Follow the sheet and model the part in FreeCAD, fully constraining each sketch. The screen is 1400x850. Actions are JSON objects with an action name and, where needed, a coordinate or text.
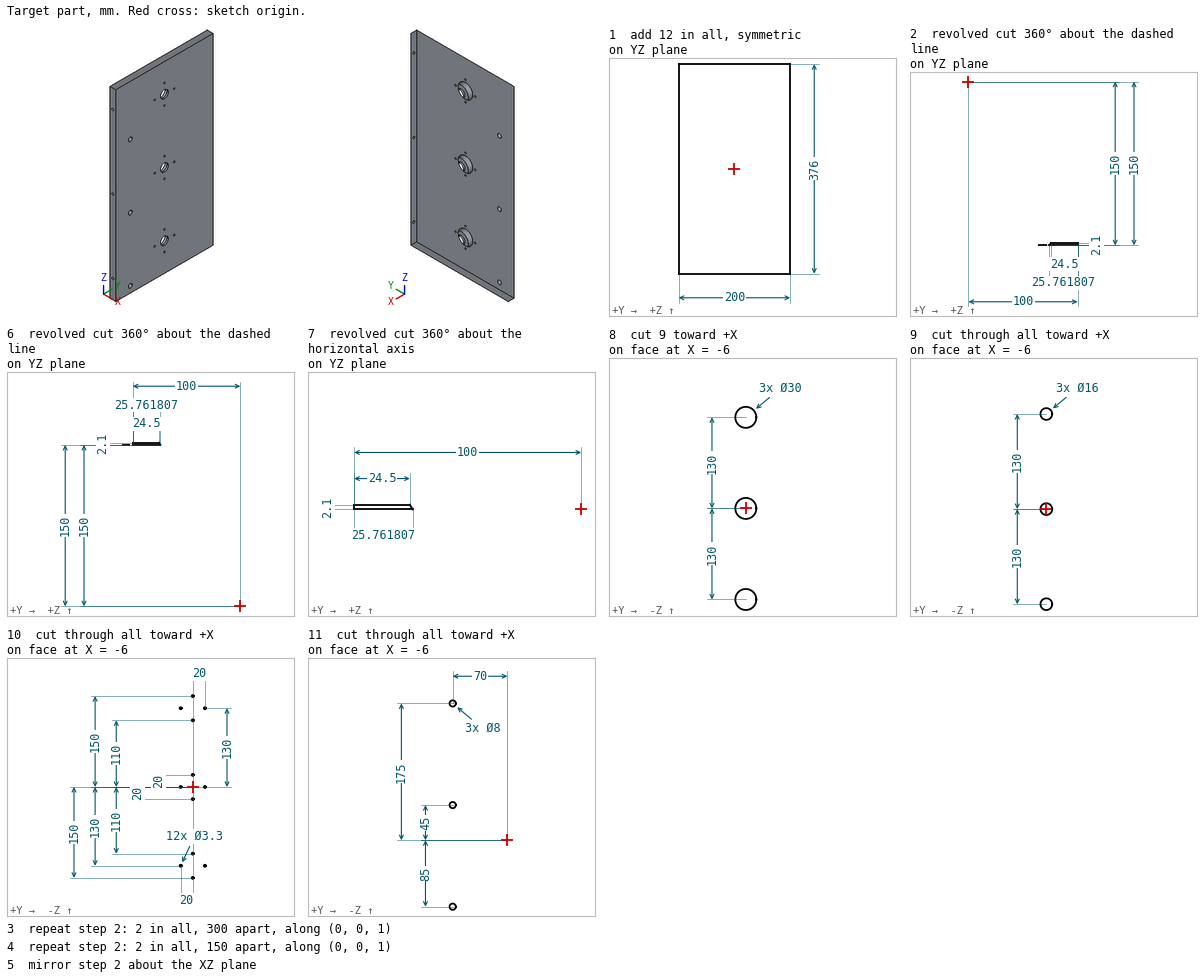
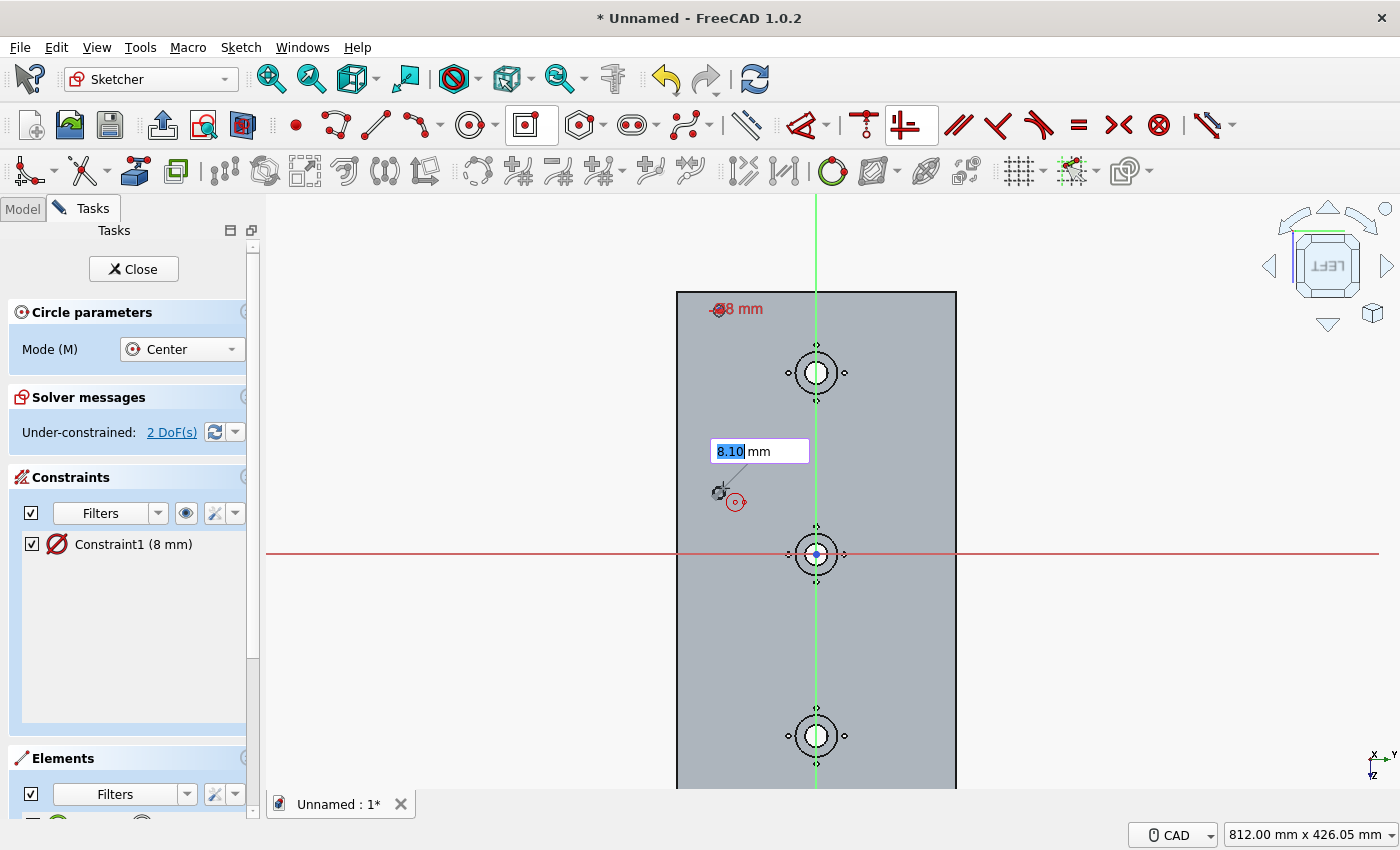
{"action": "type", "text": "8"}
{"action": "key", "text": "Return"}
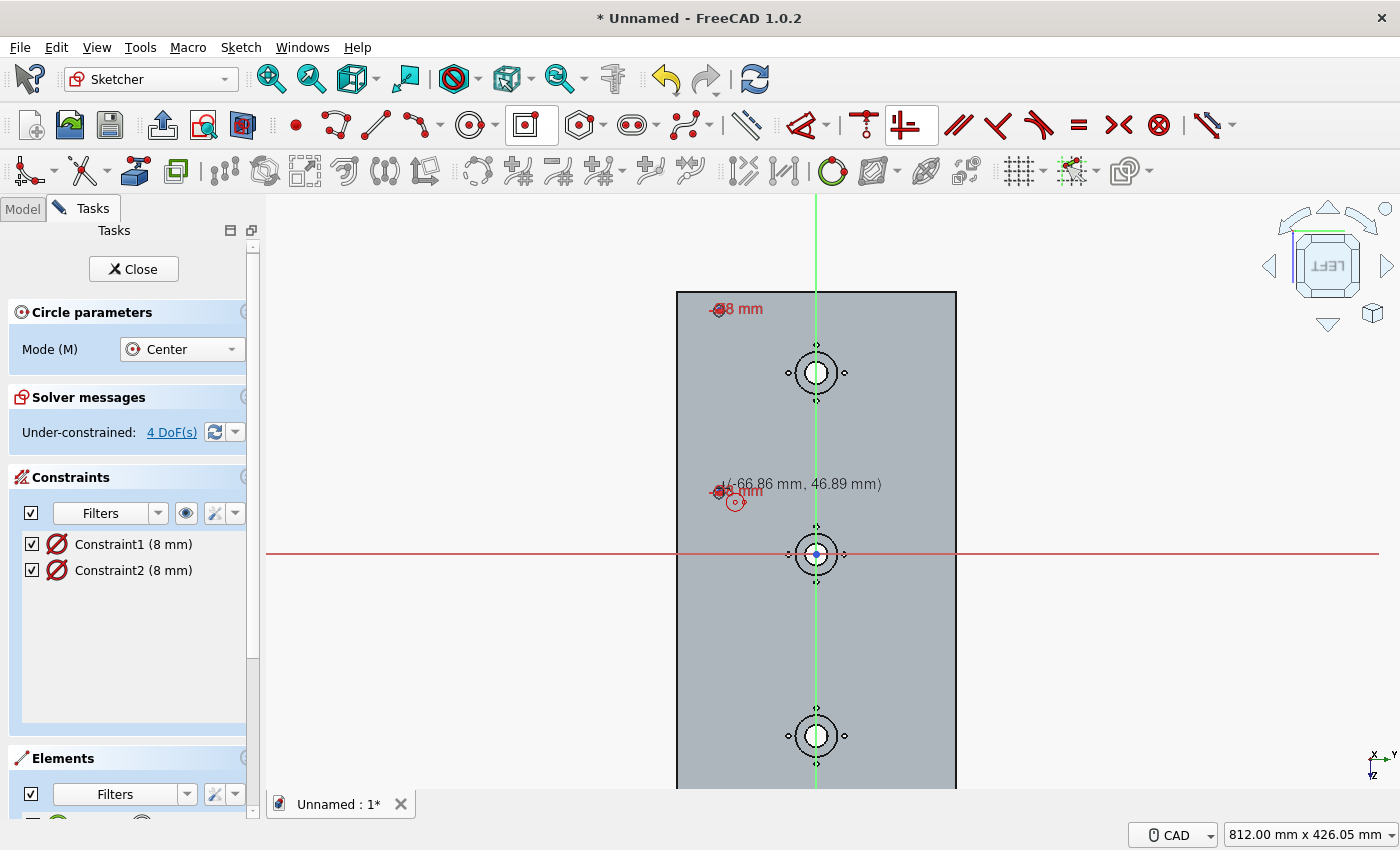
{"action": "scroll", "coordinate": [719, 673], "scroll_direction": "up", "scroll_amount": 8}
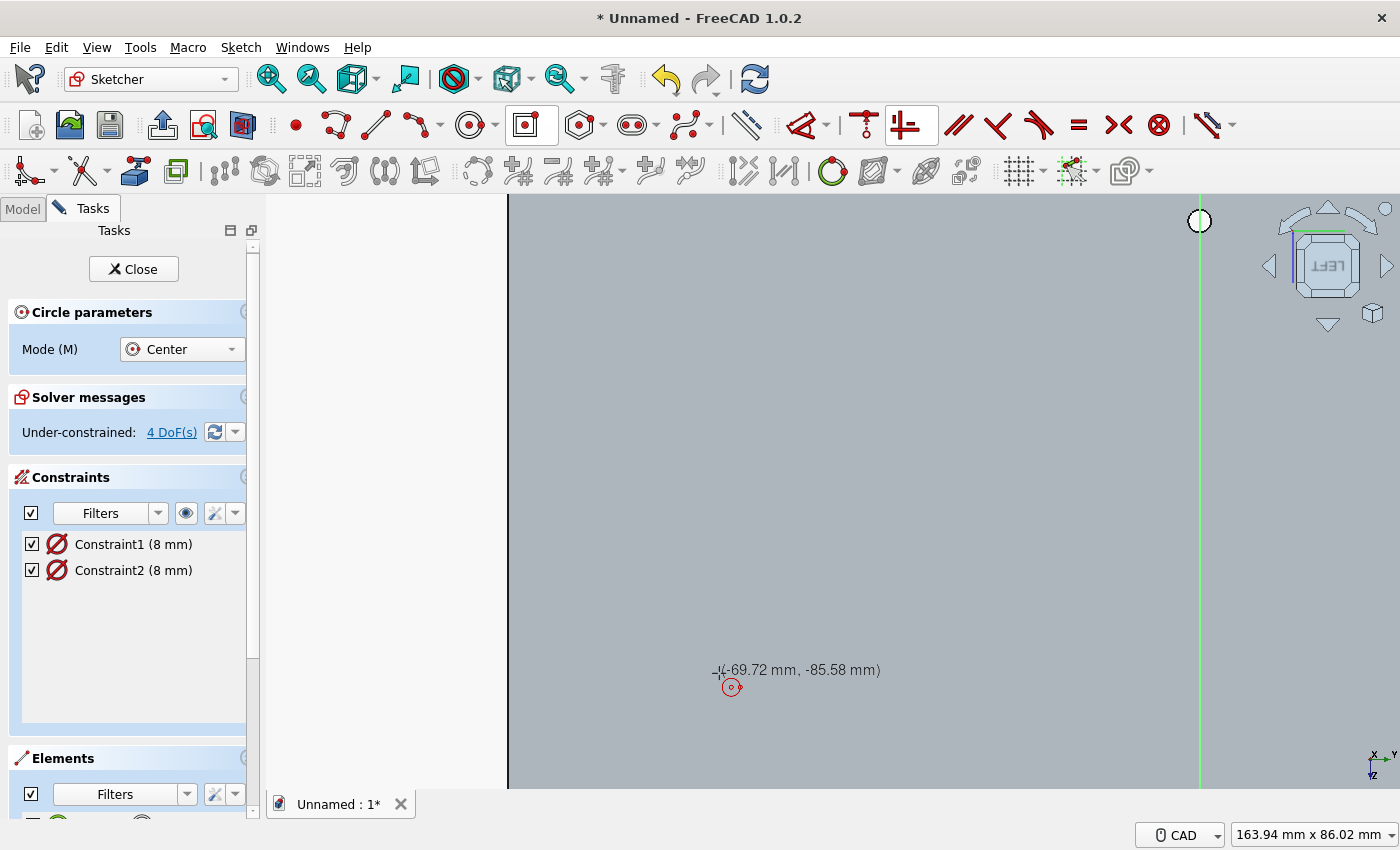
{"action": "scroll", "coordinate": [719, 674], "scroll_direction": "down", "scroll_amount": 8}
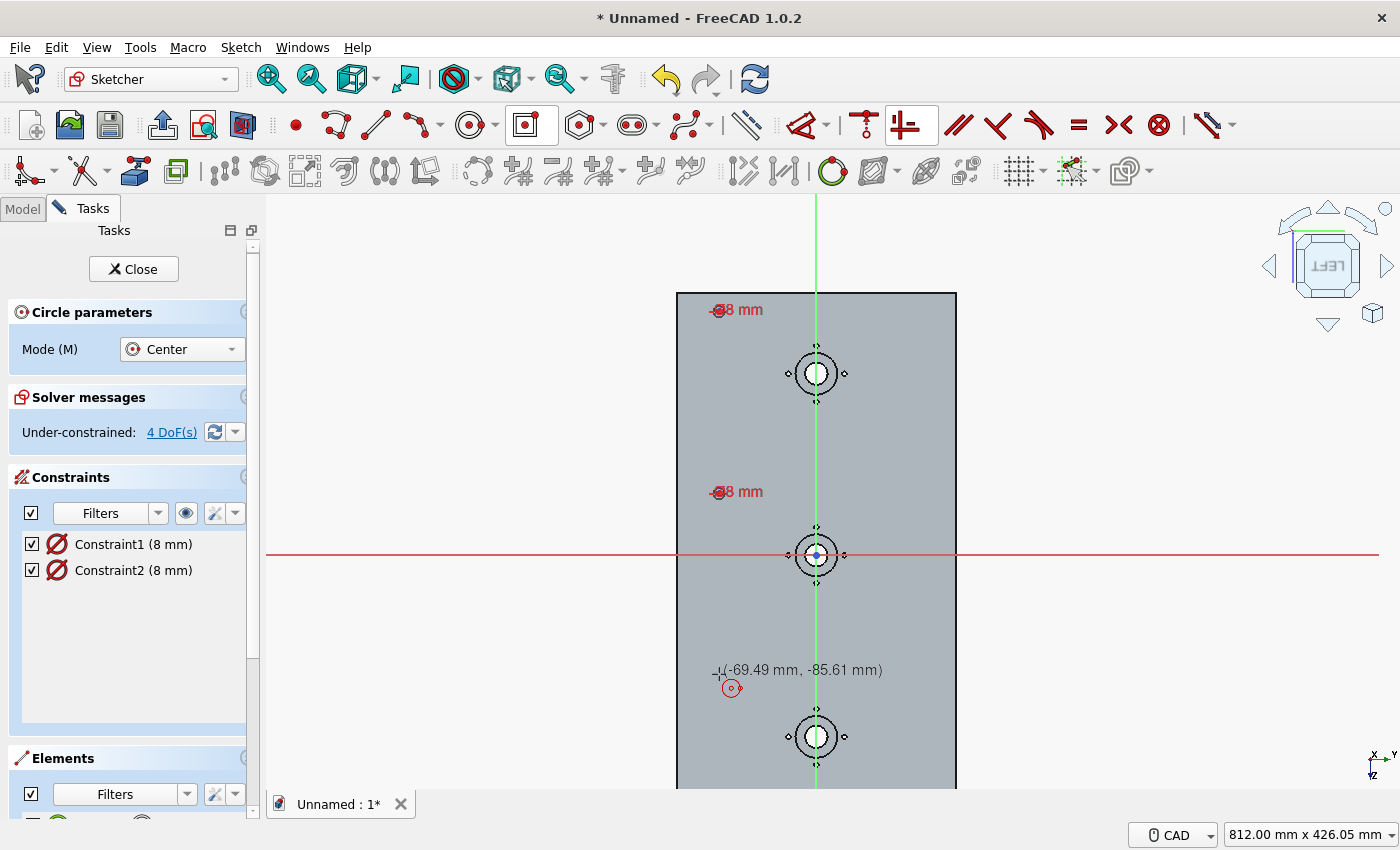
{"action": "left_click", "coordinate": [719, 674]}
{"action": "mouse_move", "coordinate": [723, 670]}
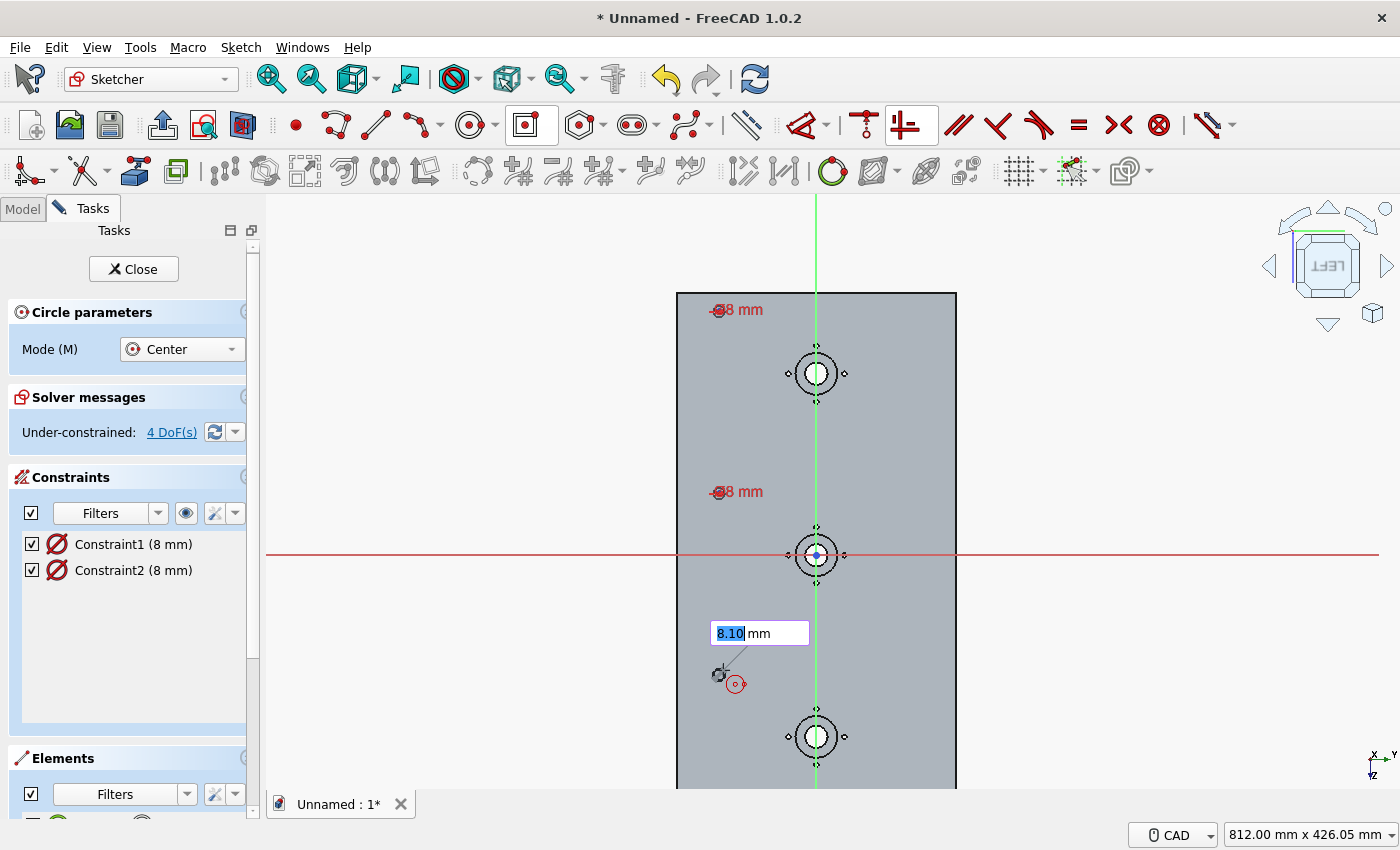
{"action": "type", "text": "8"}
{"action": "key", "text": "Return"}
{"action": "key", "text": "Escape"}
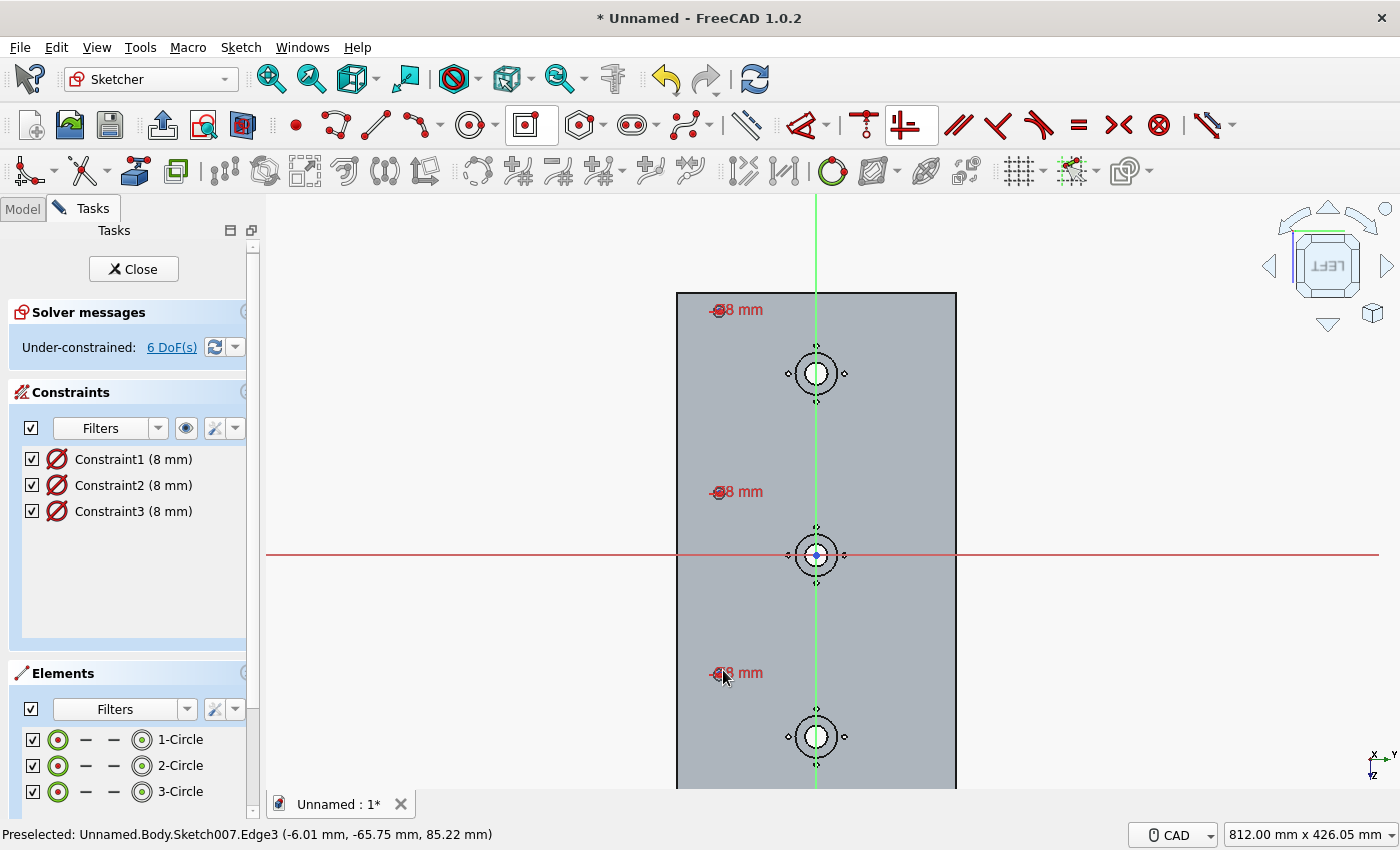
{"action": "left_click", "coordinate": [719, 312]}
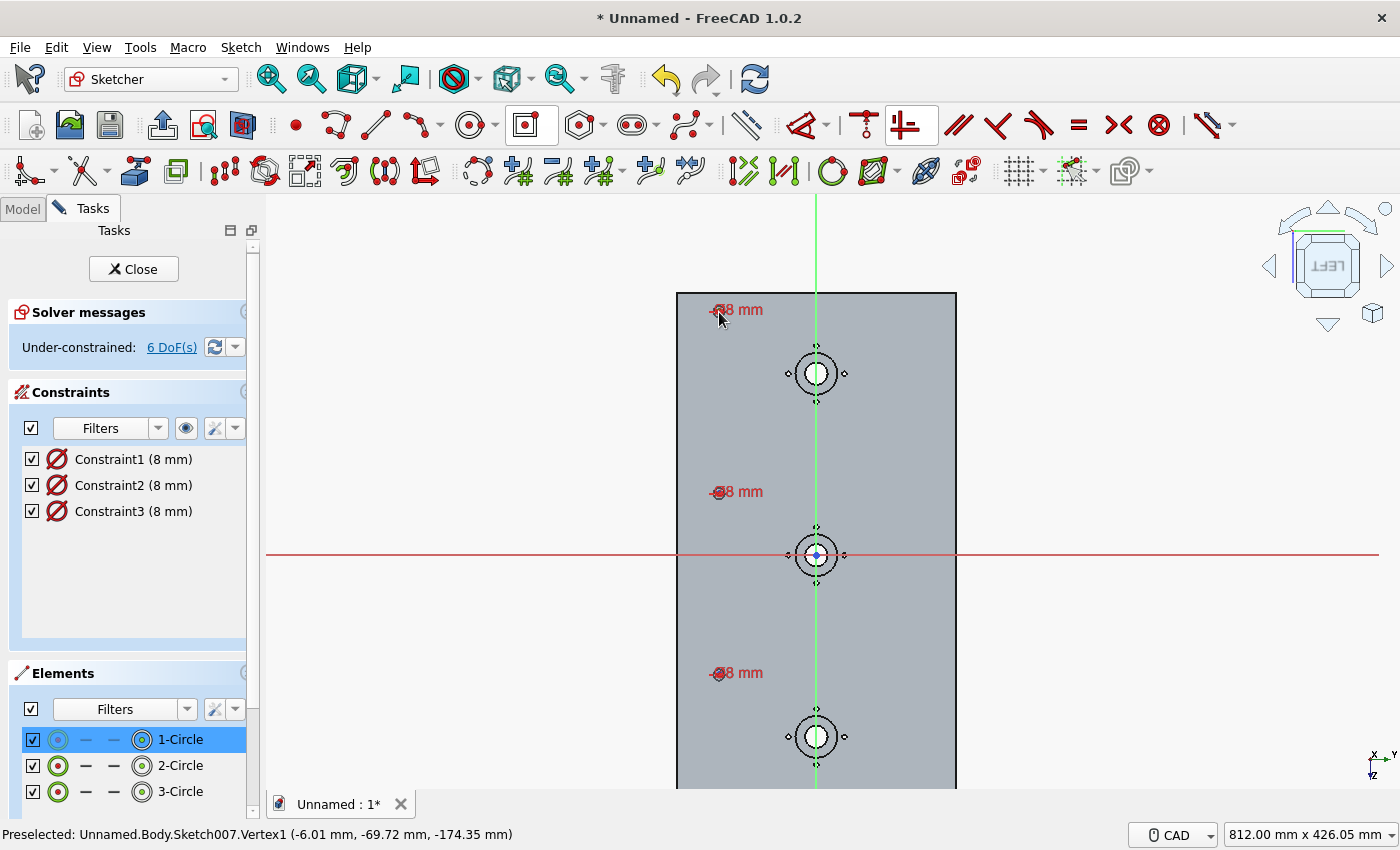
{"action": "left_click", "coordinate": [719, 494]}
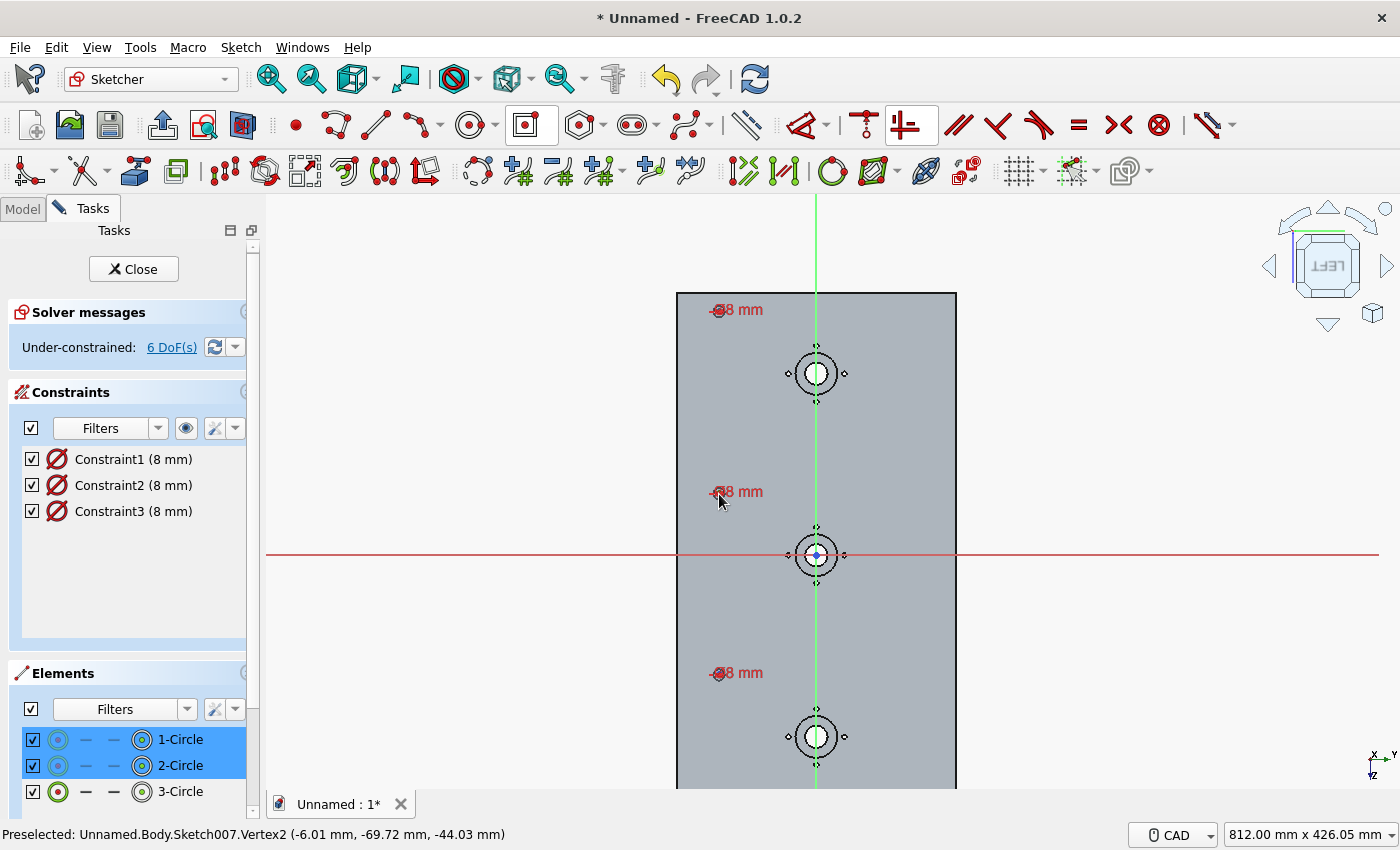
{"action": "left_click", "coordinate": [932, 126]}